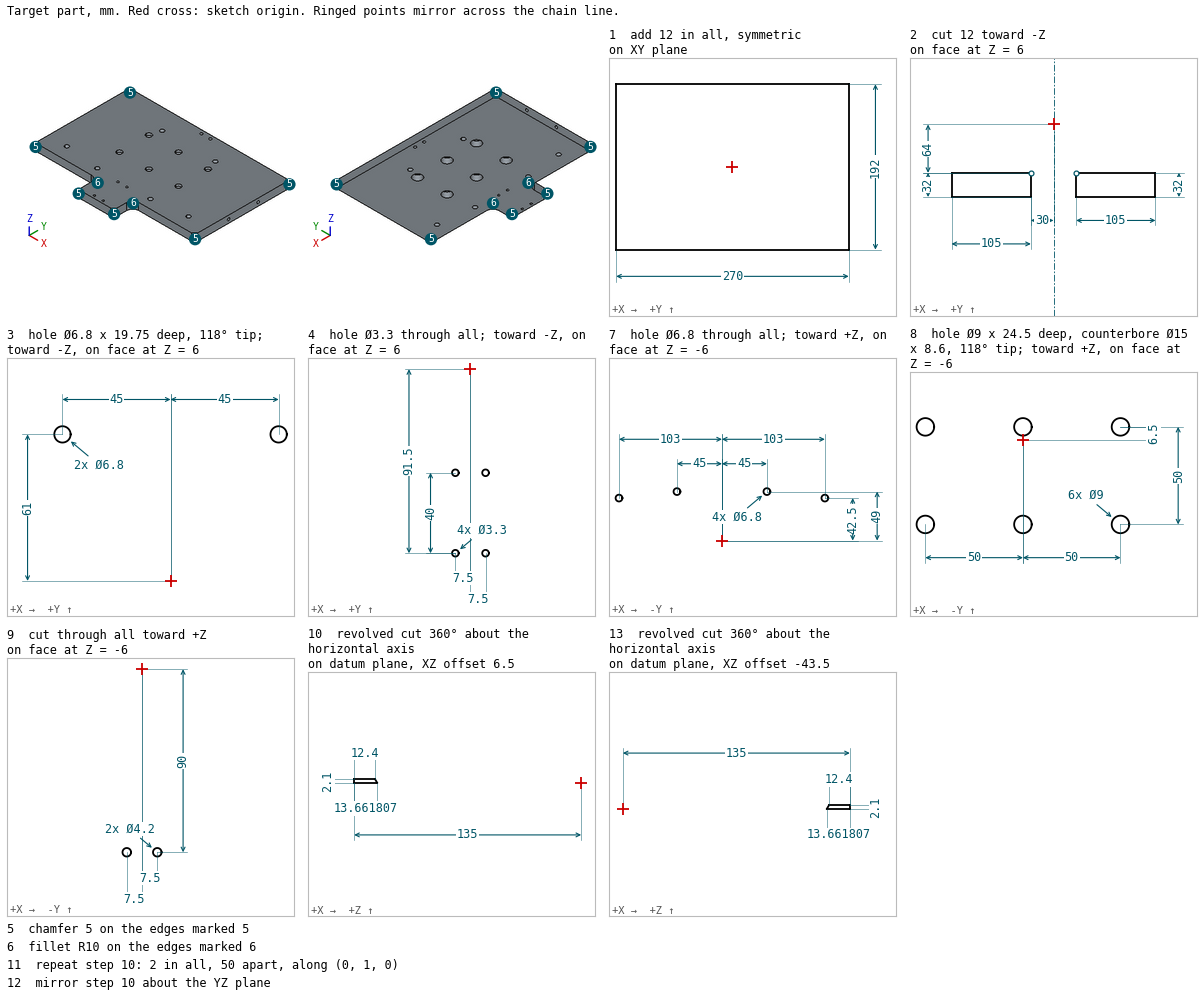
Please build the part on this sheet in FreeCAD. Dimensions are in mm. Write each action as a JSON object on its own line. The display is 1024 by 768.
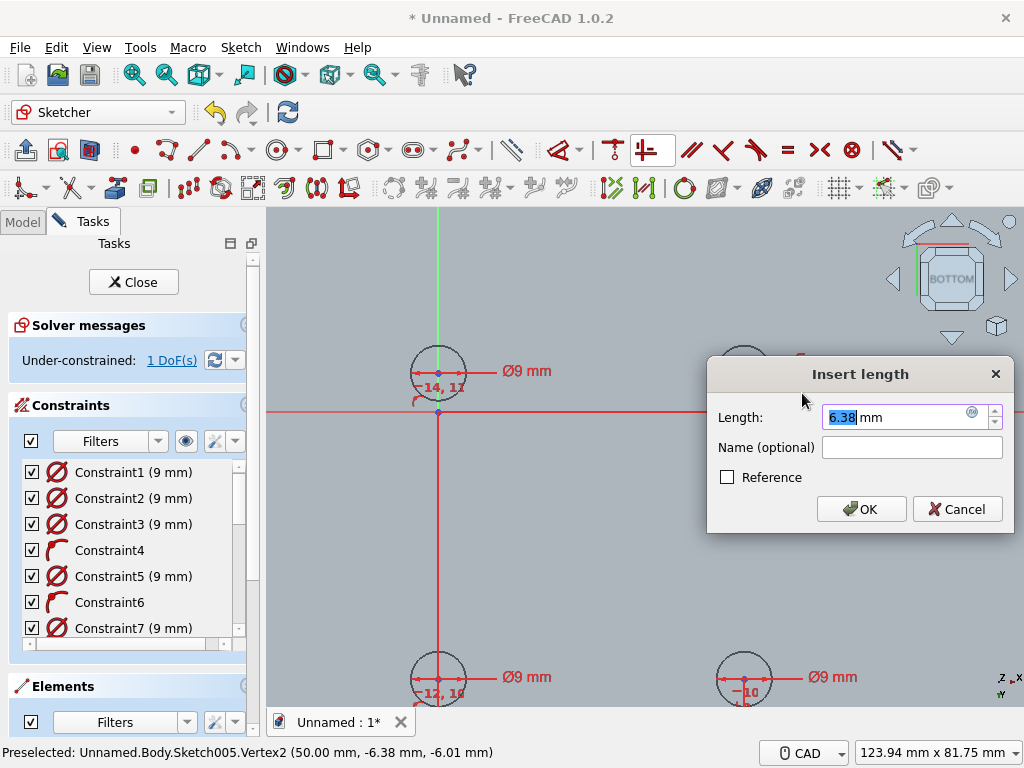
{"action": "type", "text": "6.5"}
{"action": "key", "text": "Return"}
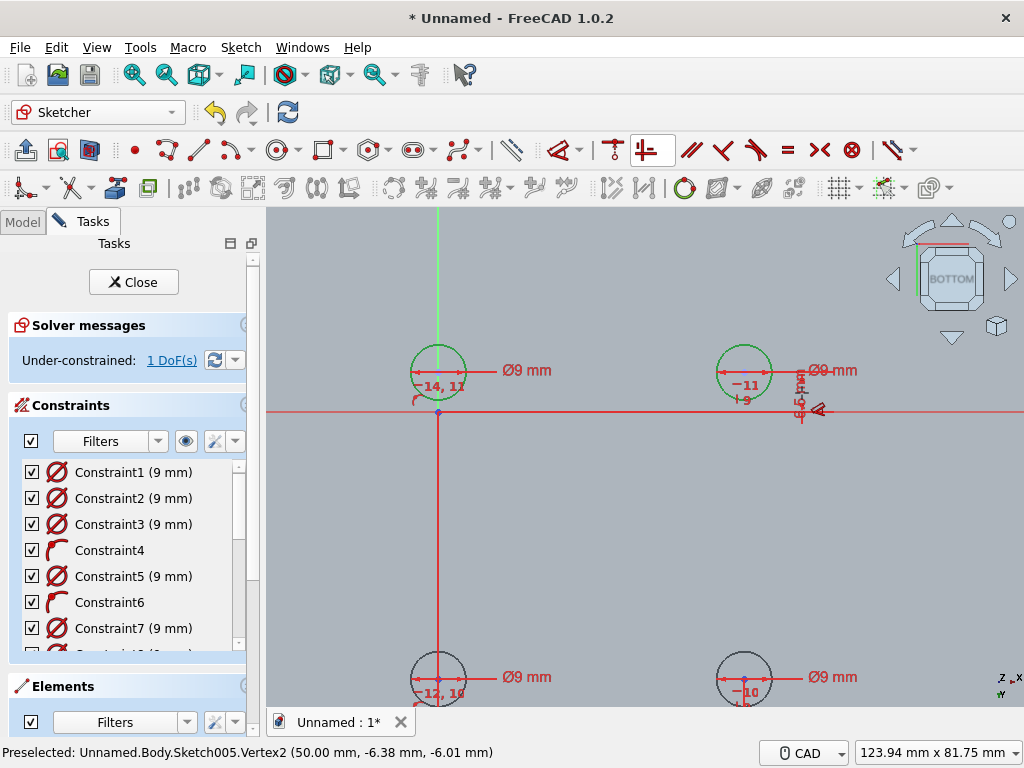
{"action": "scroll", "coordinate": [744, 374], "scroll_direction": "down", "scroll_amount": 3}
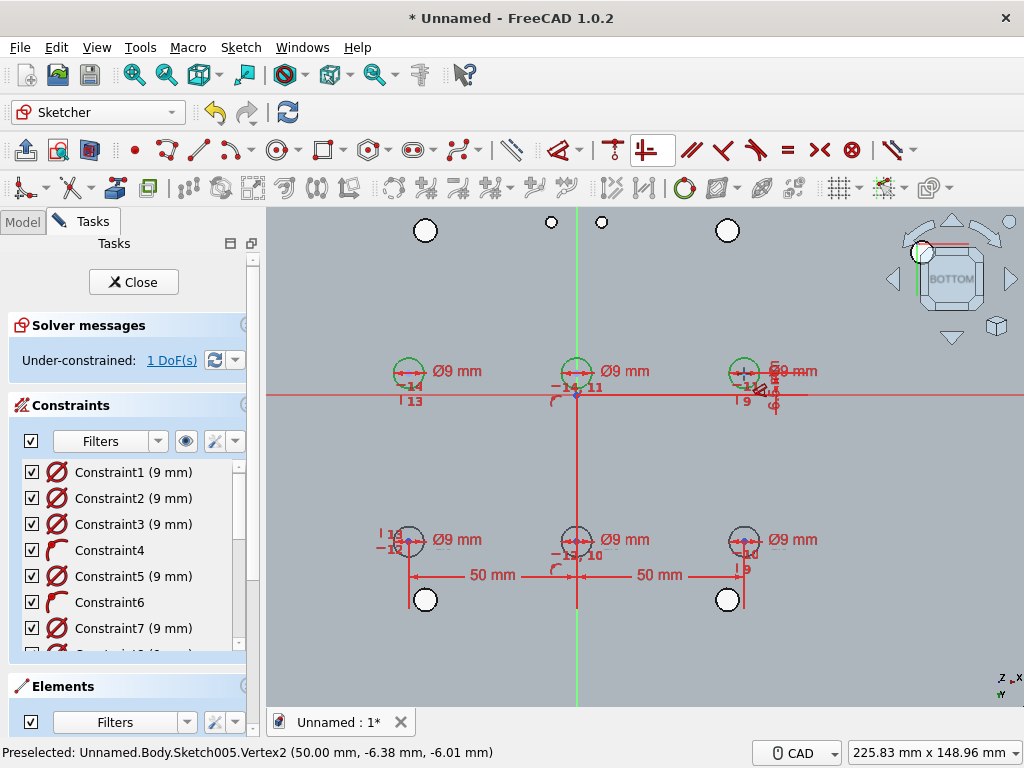
{"action": "left_click", "coordinate": [744, 542]}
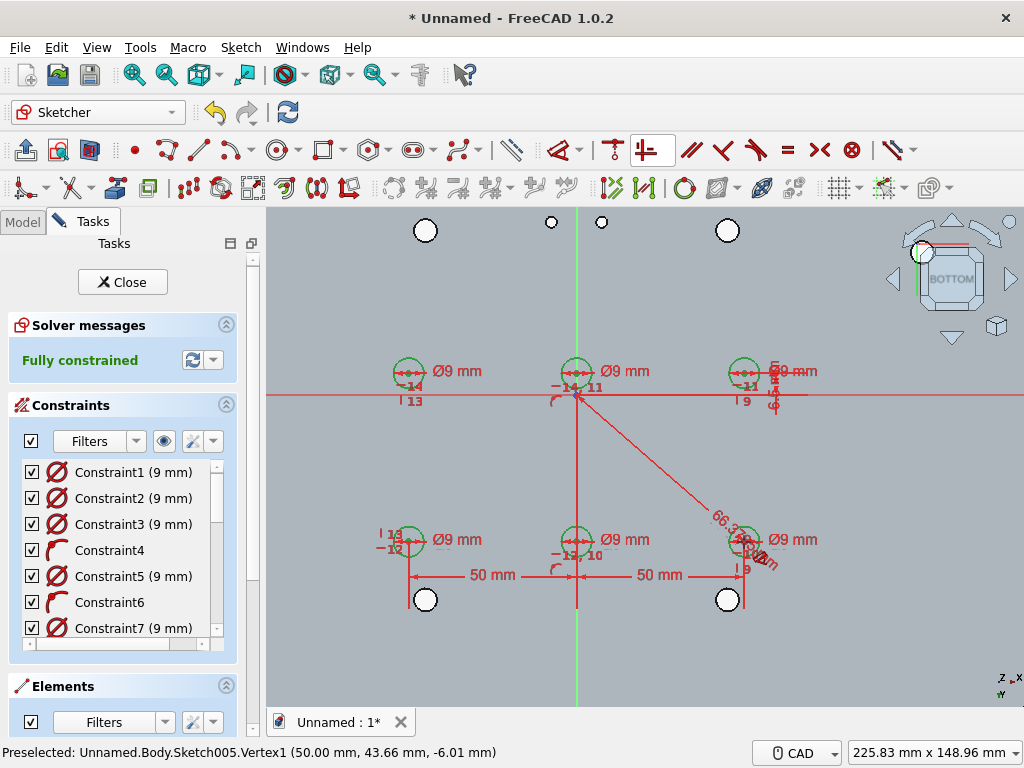
{"action": "left_click", "coordinate": [744, 373]}
{"action": "left_click", "coordinate": [778, 457]}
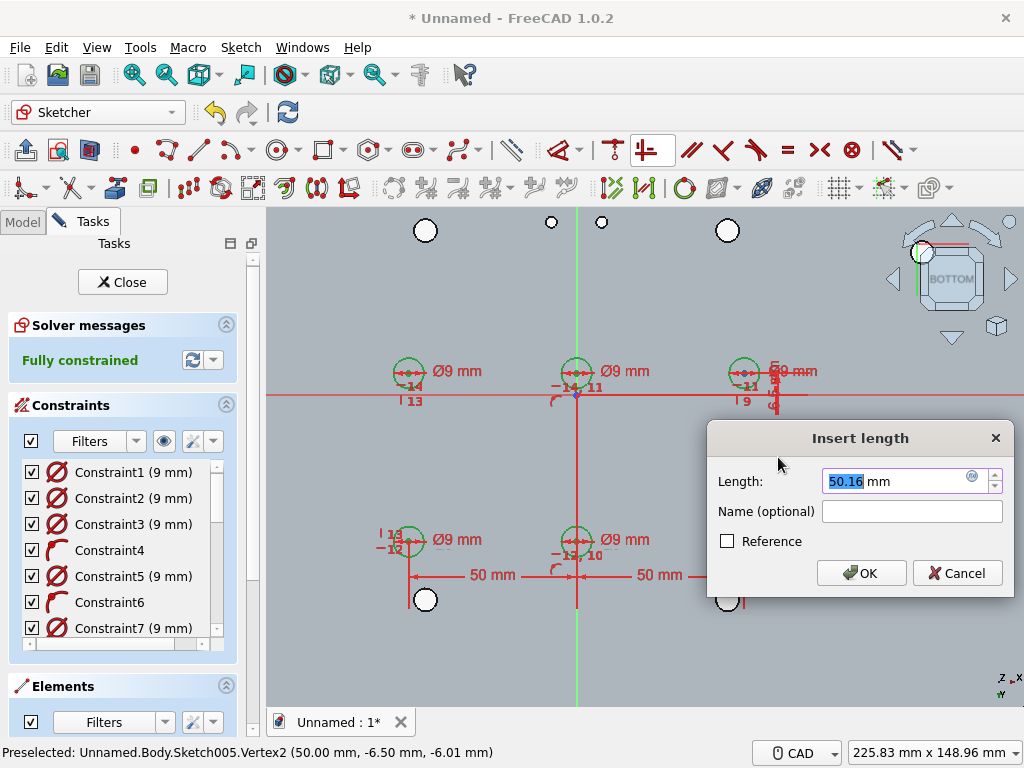
{"action": "type", "text": "50"}
{"action": "key", "text": "Return"}
{"action": "key", "text": "Escape"}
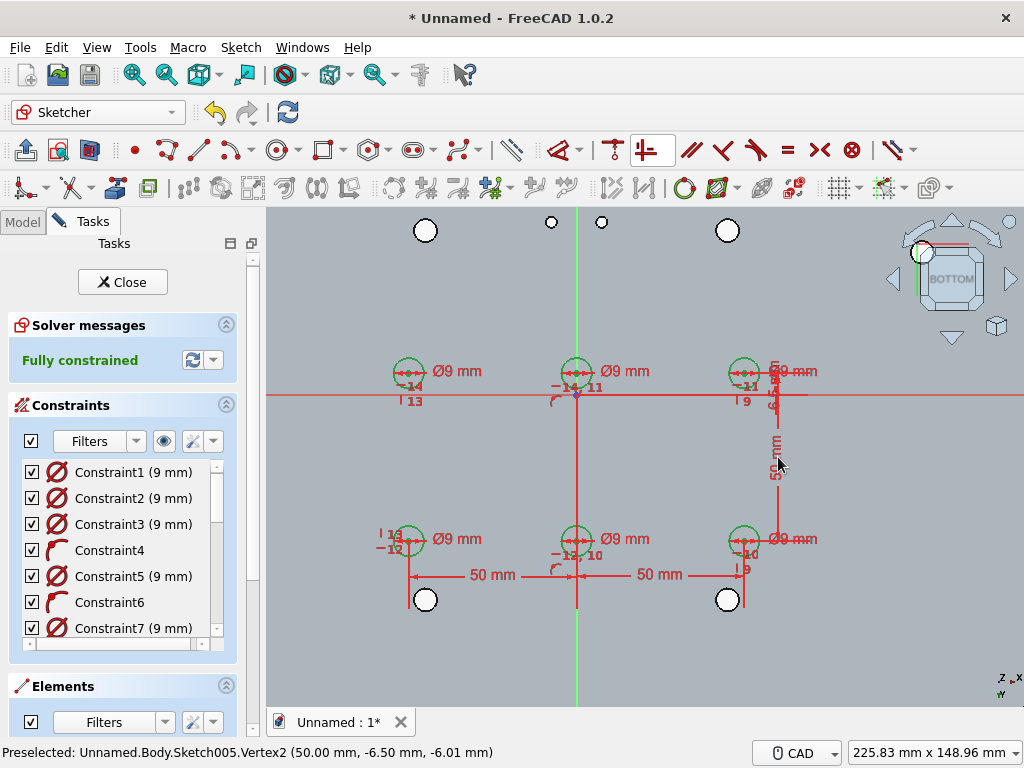
{"action": "left_click", "coordinate": [123, 282]}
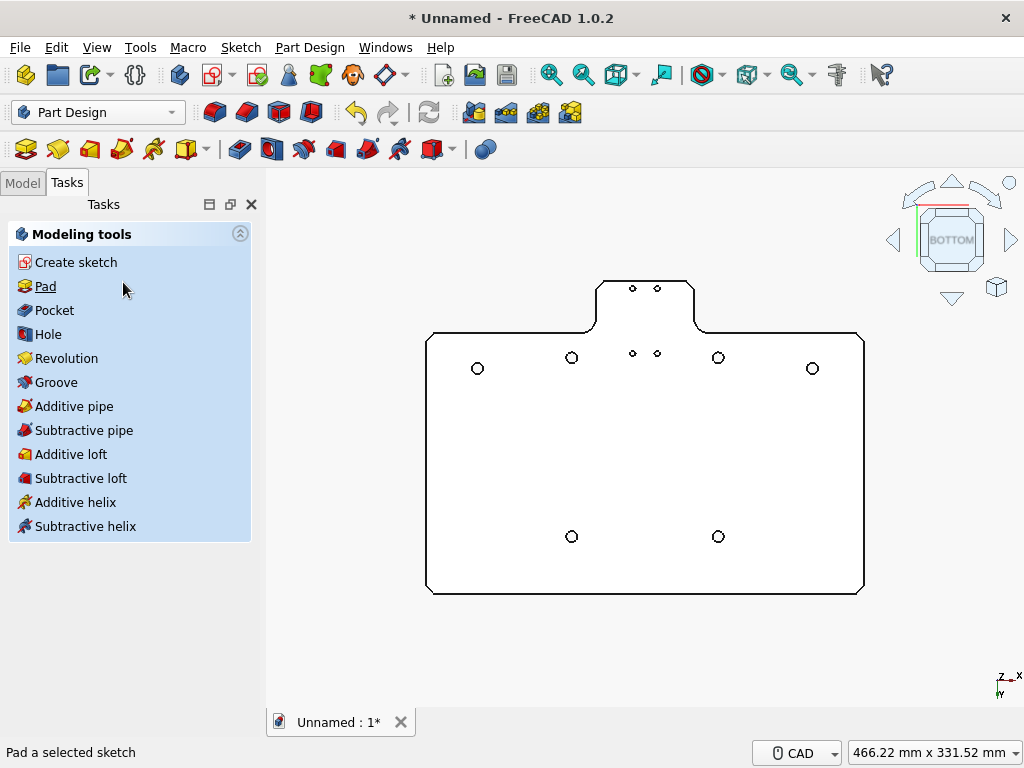
{"action": "left_click", "coordinate": [272, 150]}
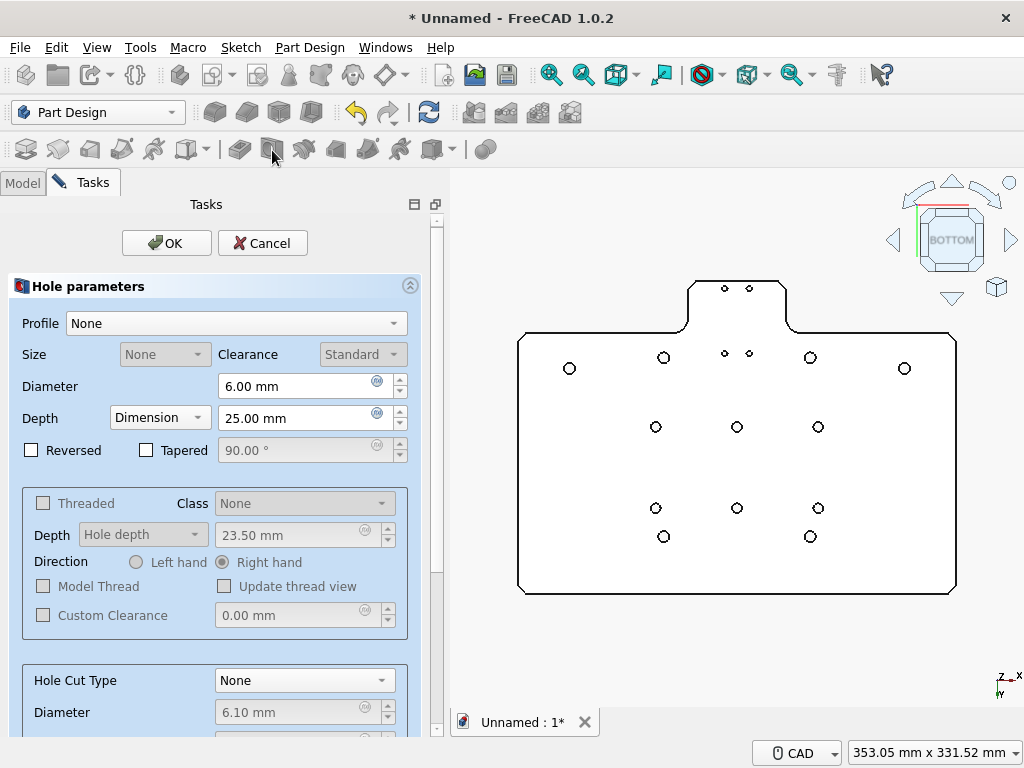
{"action": "triple_click", "coordinate": [305, 386]}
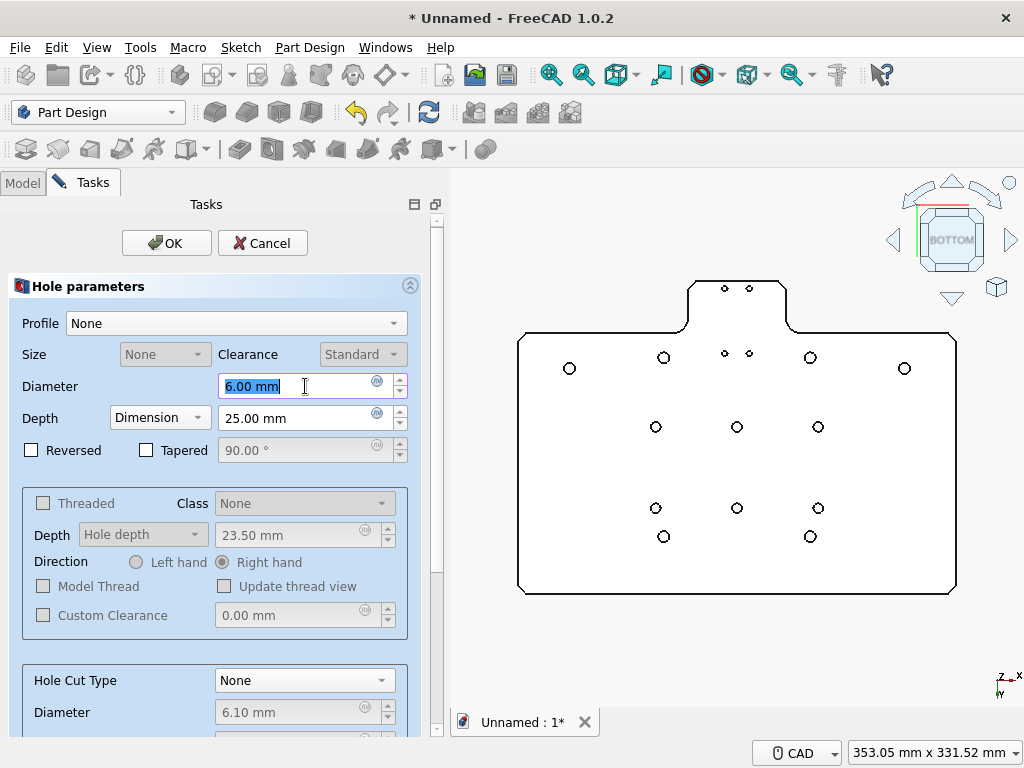
{"action": "type", "text": "9"}
{"action": "key", "text": "Tab"}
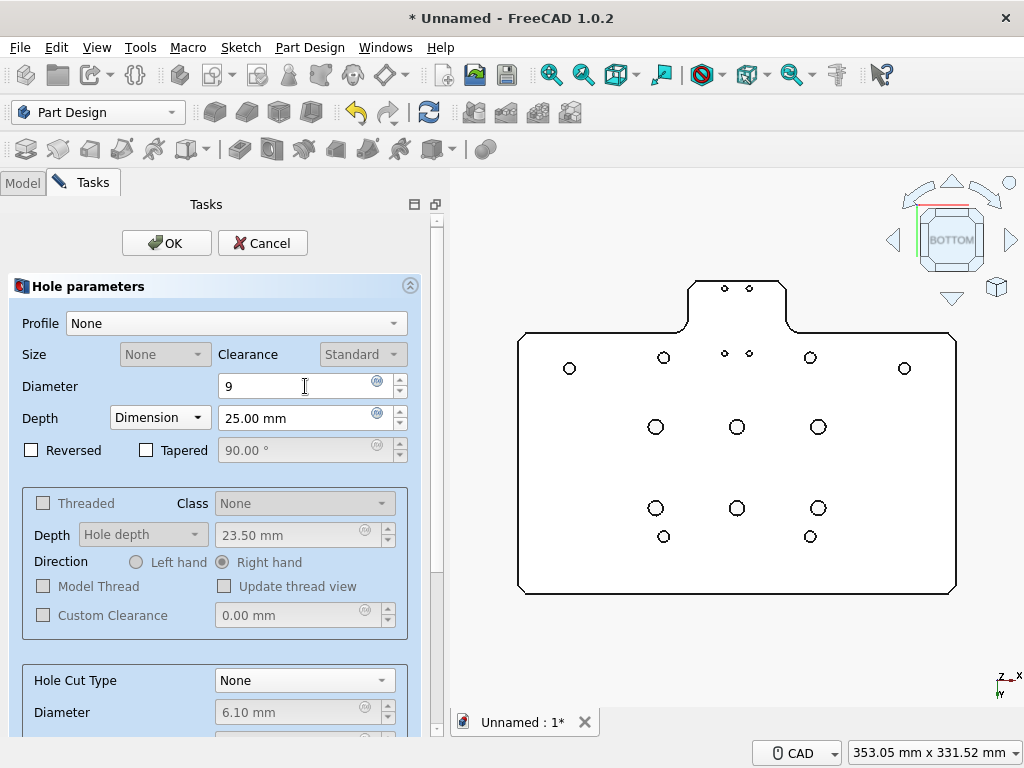
{"action": "triple_click", "coordinate": [305, 418]}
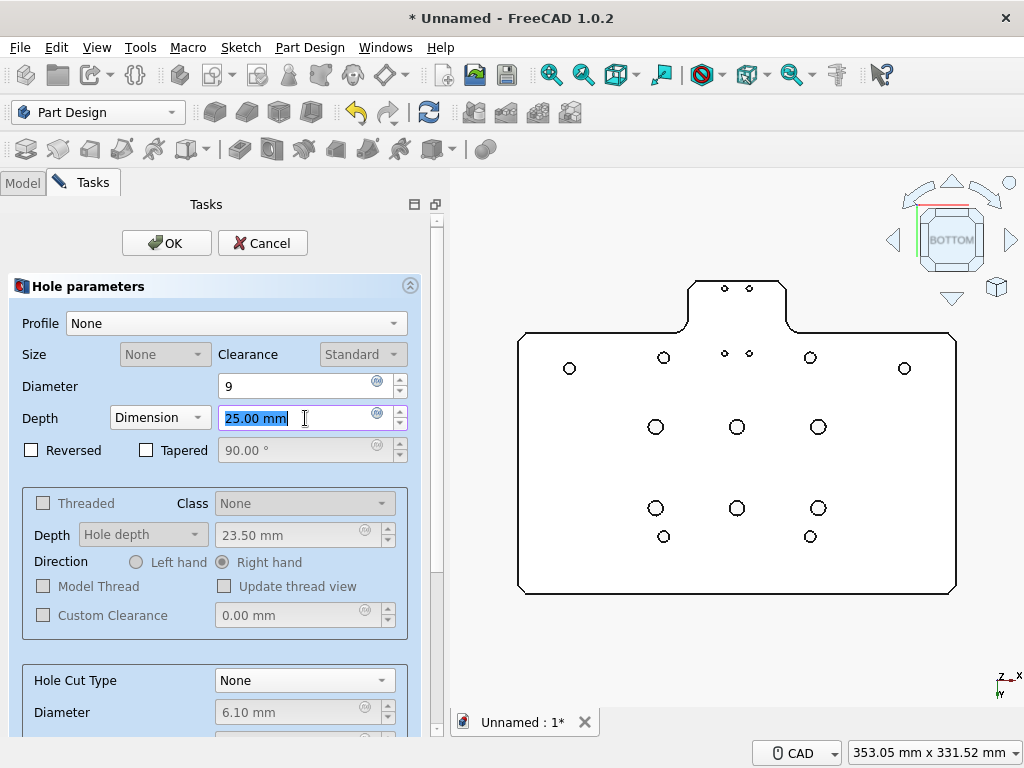
{"action": "type", "text": "24.5"}
{"action": "key", "text": "Tab"}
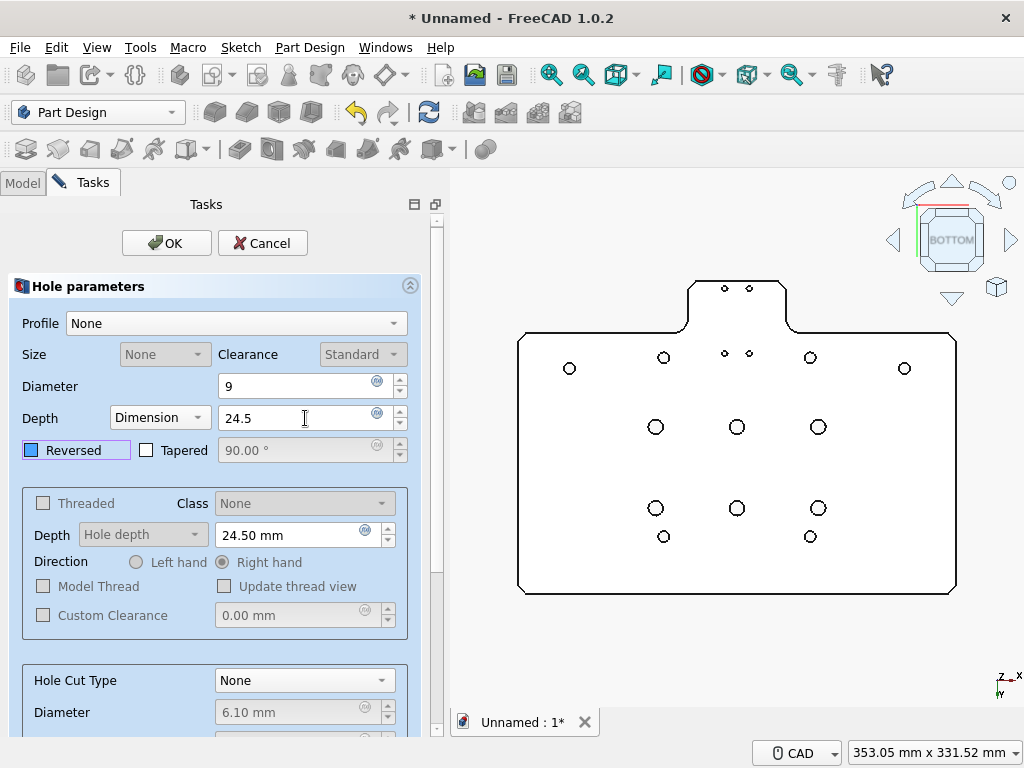
{"action": "left_click", "coordinate": [306, 680]}